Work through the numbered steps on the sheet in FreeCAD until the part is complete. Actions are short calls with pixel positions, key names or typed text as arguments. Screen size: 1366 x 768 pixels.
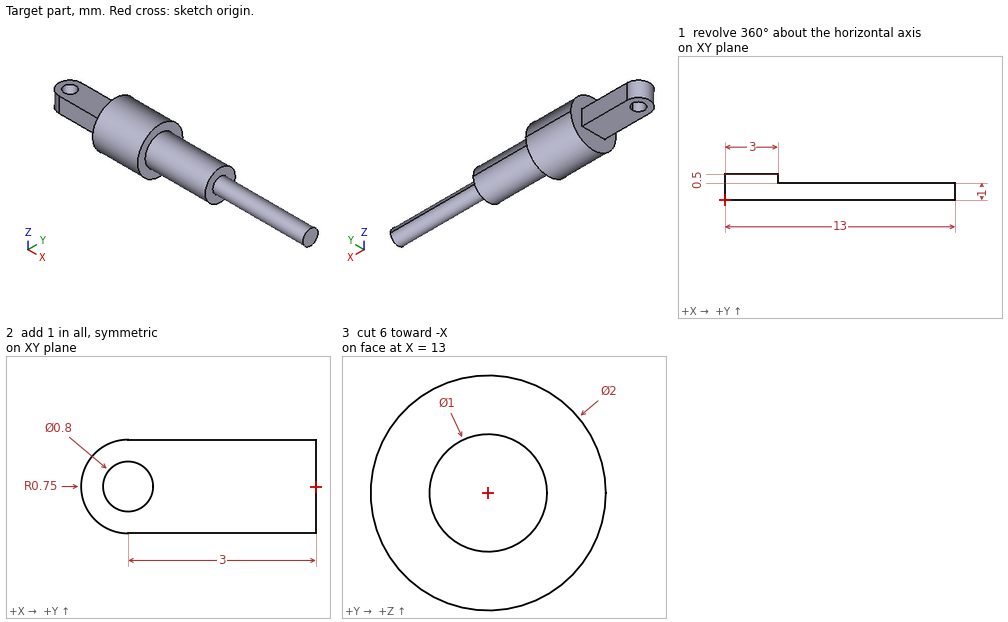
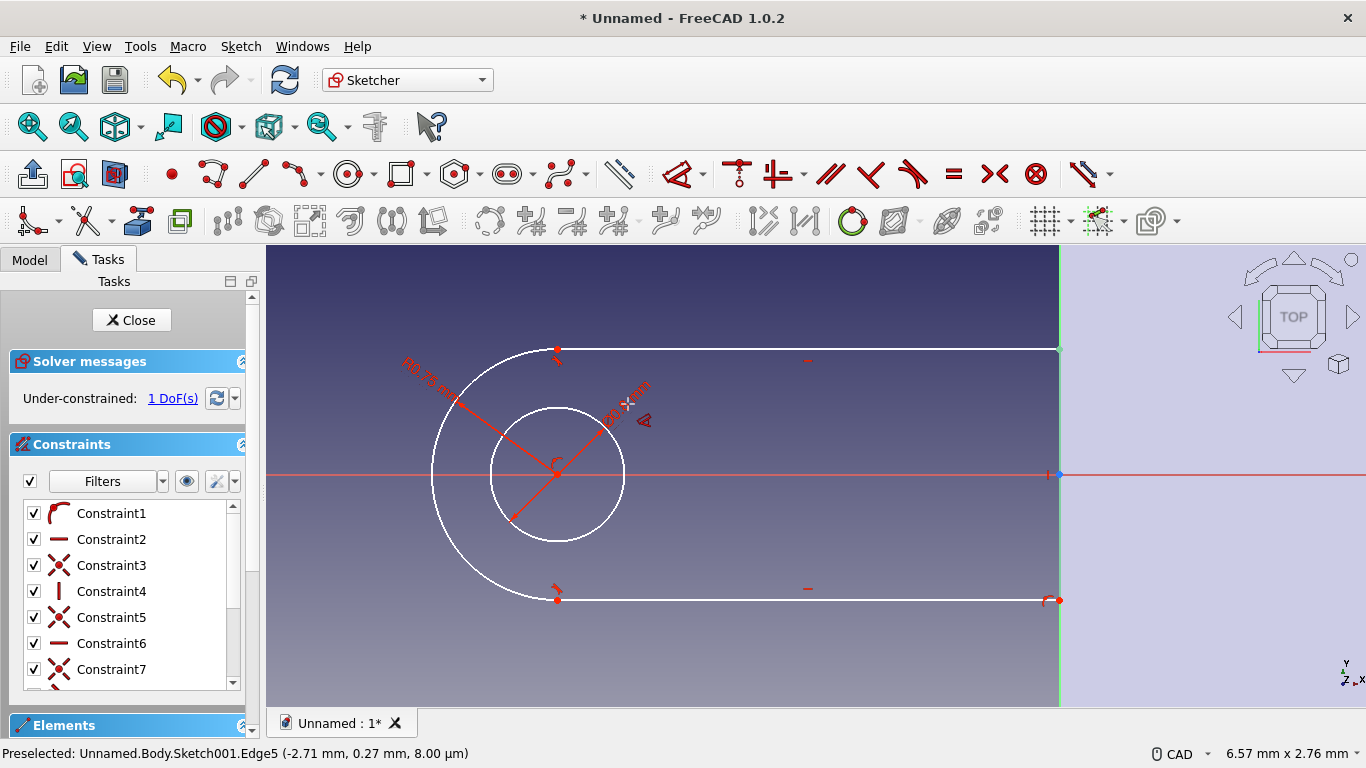
click(708, 600)
click(809, 634)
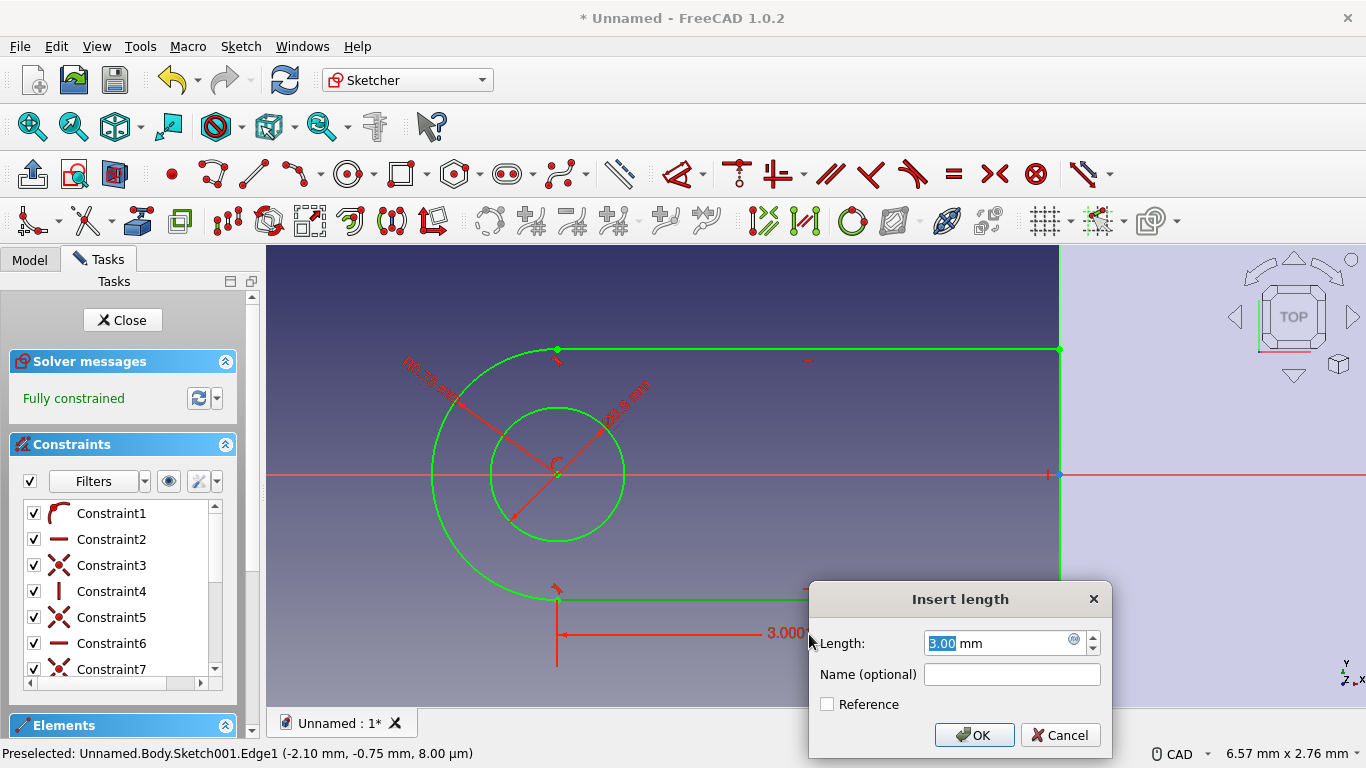
text(3)
key(Return)
key(Escape)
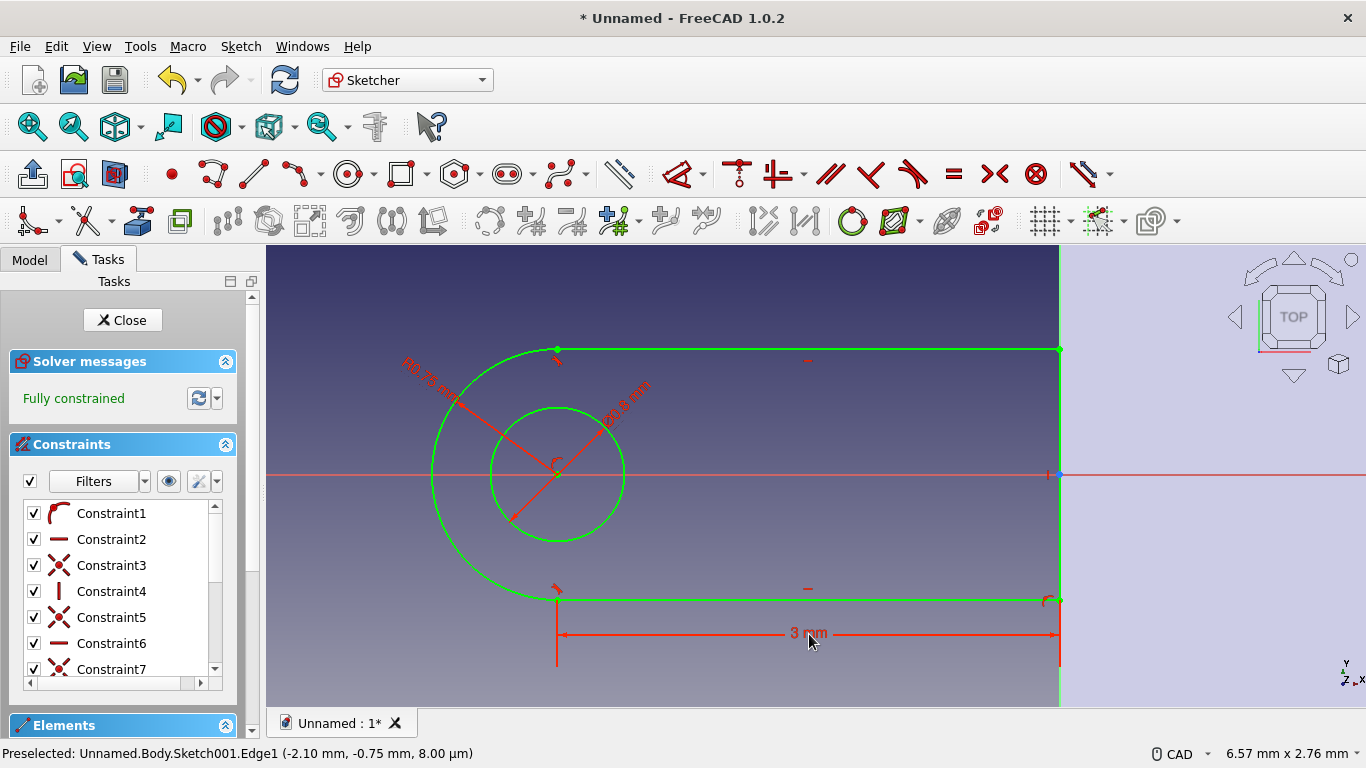
click(123, 320)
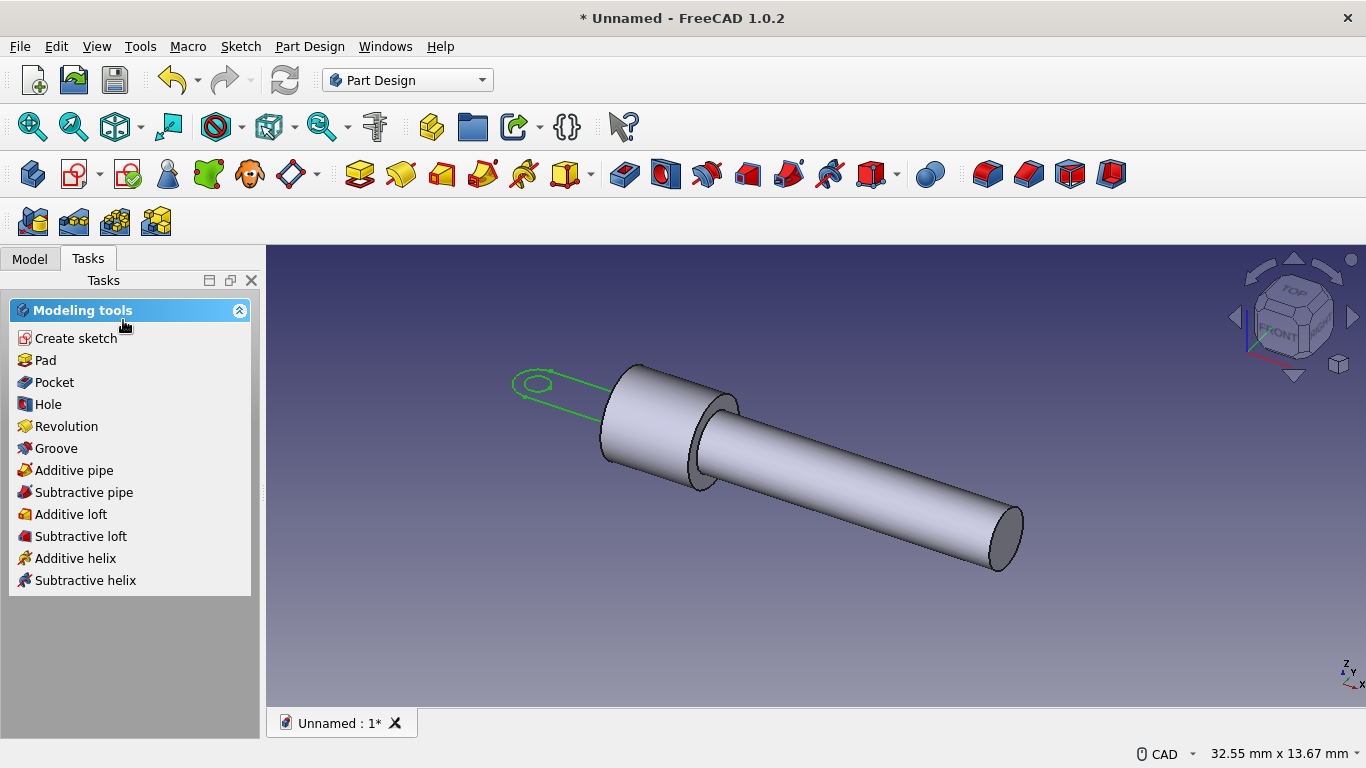
click(360, 174)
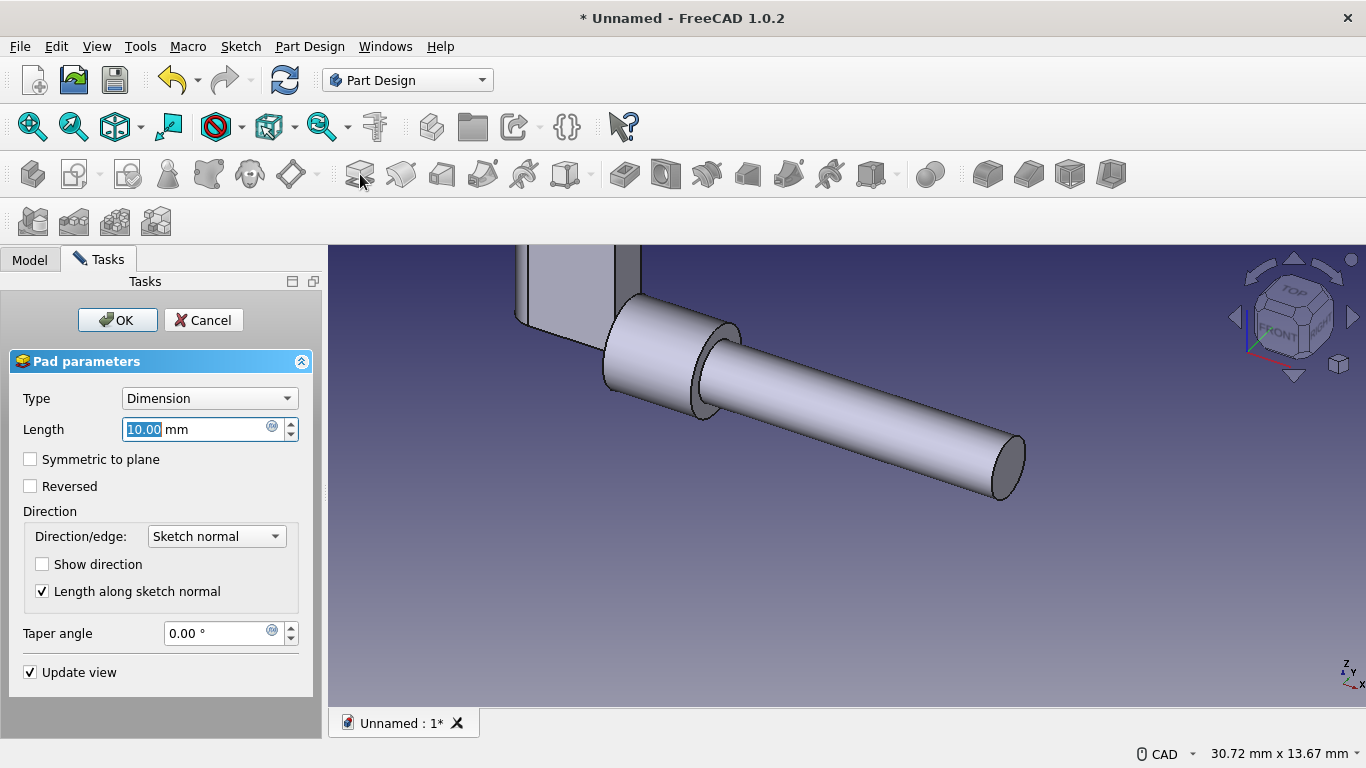
text(1)
key(Tab)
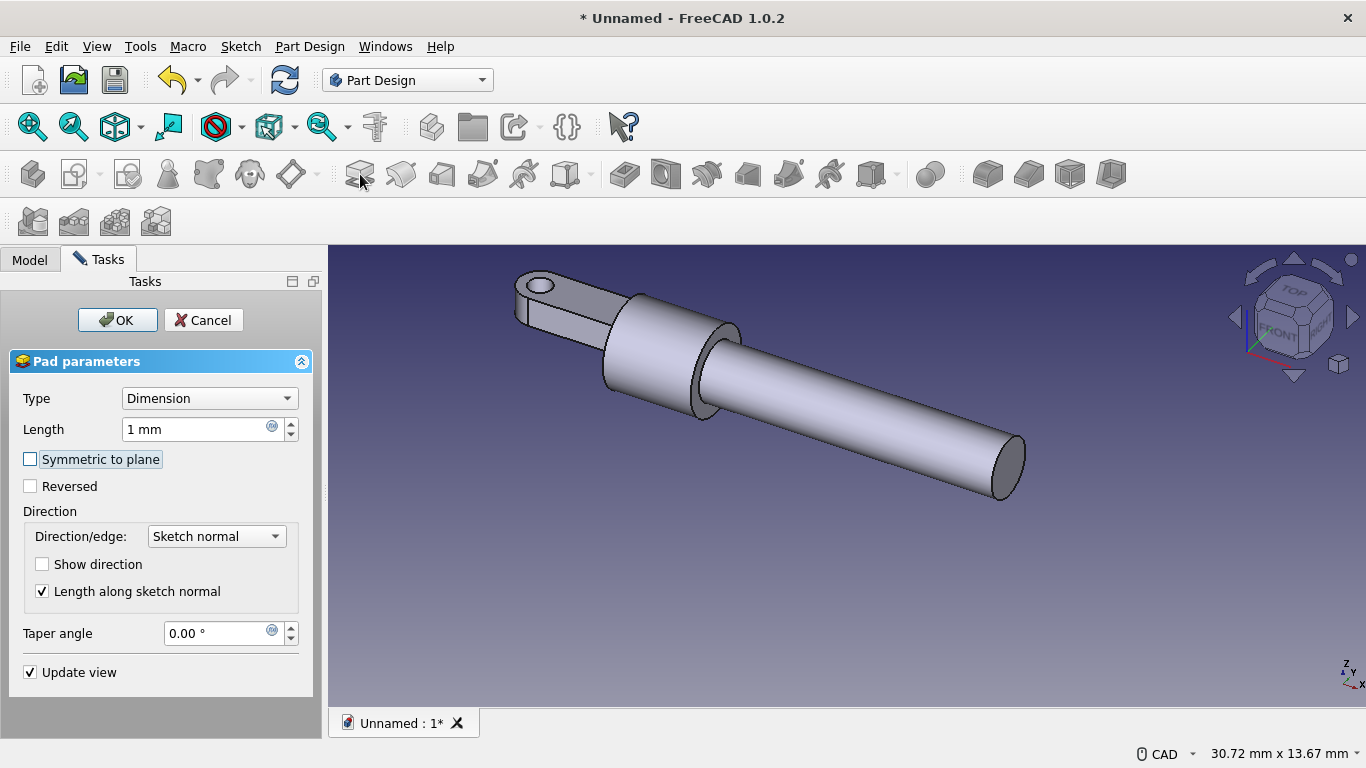
click(31, 459)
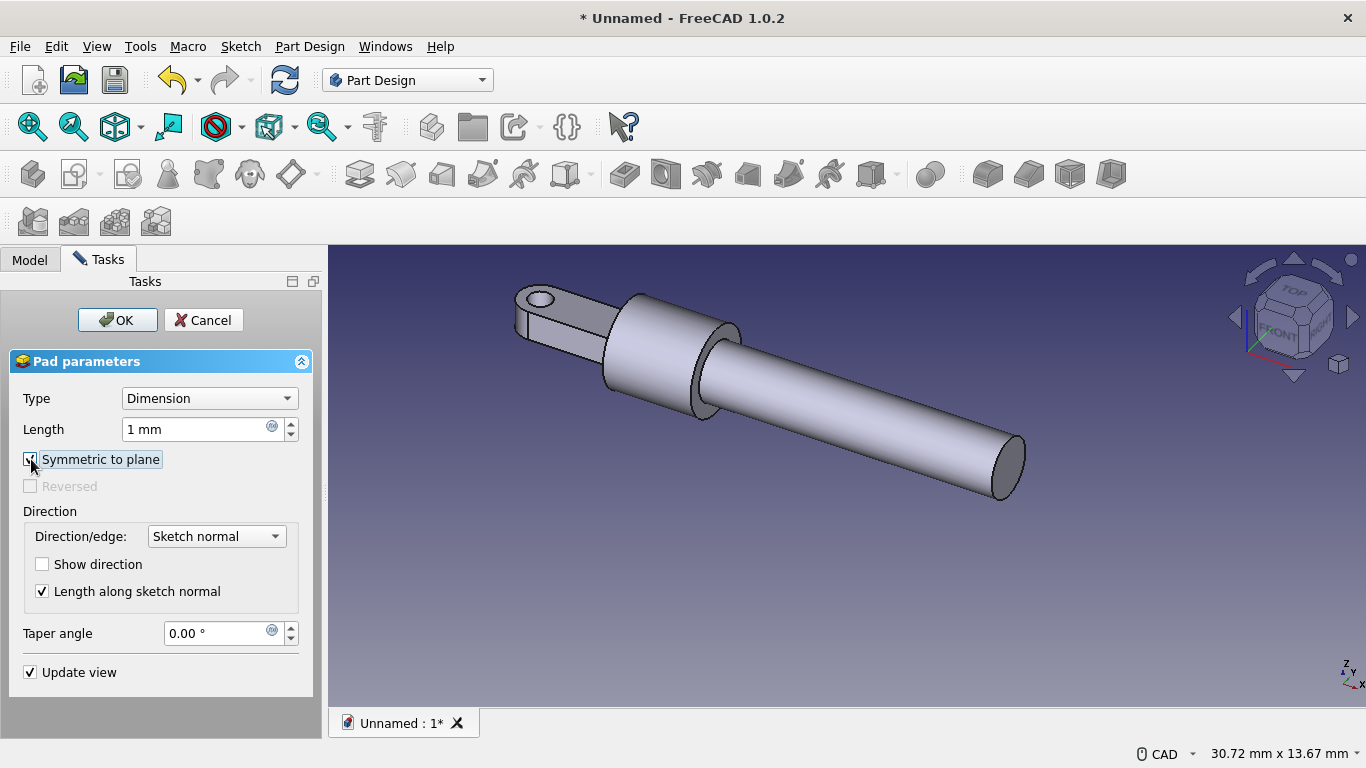
click(118, 320)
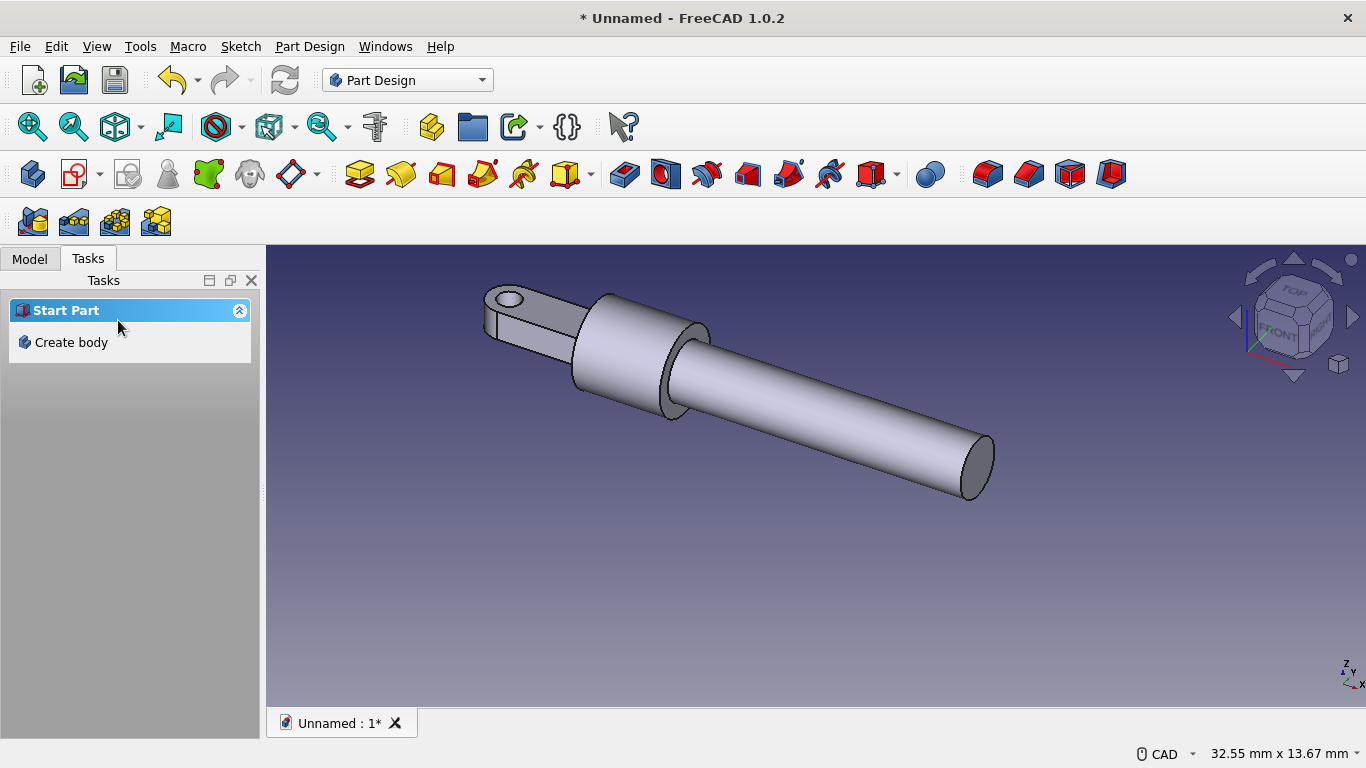
click(33, 128)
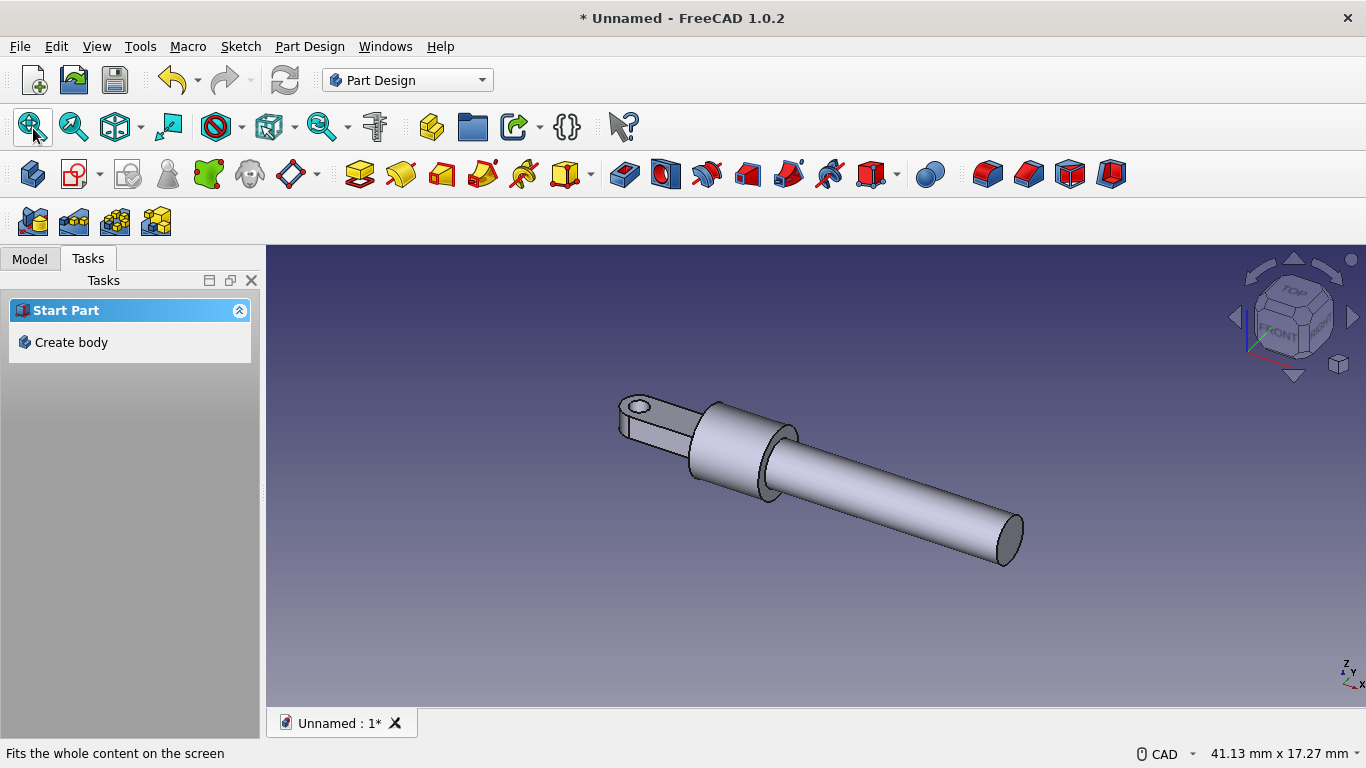
click(1010, 539)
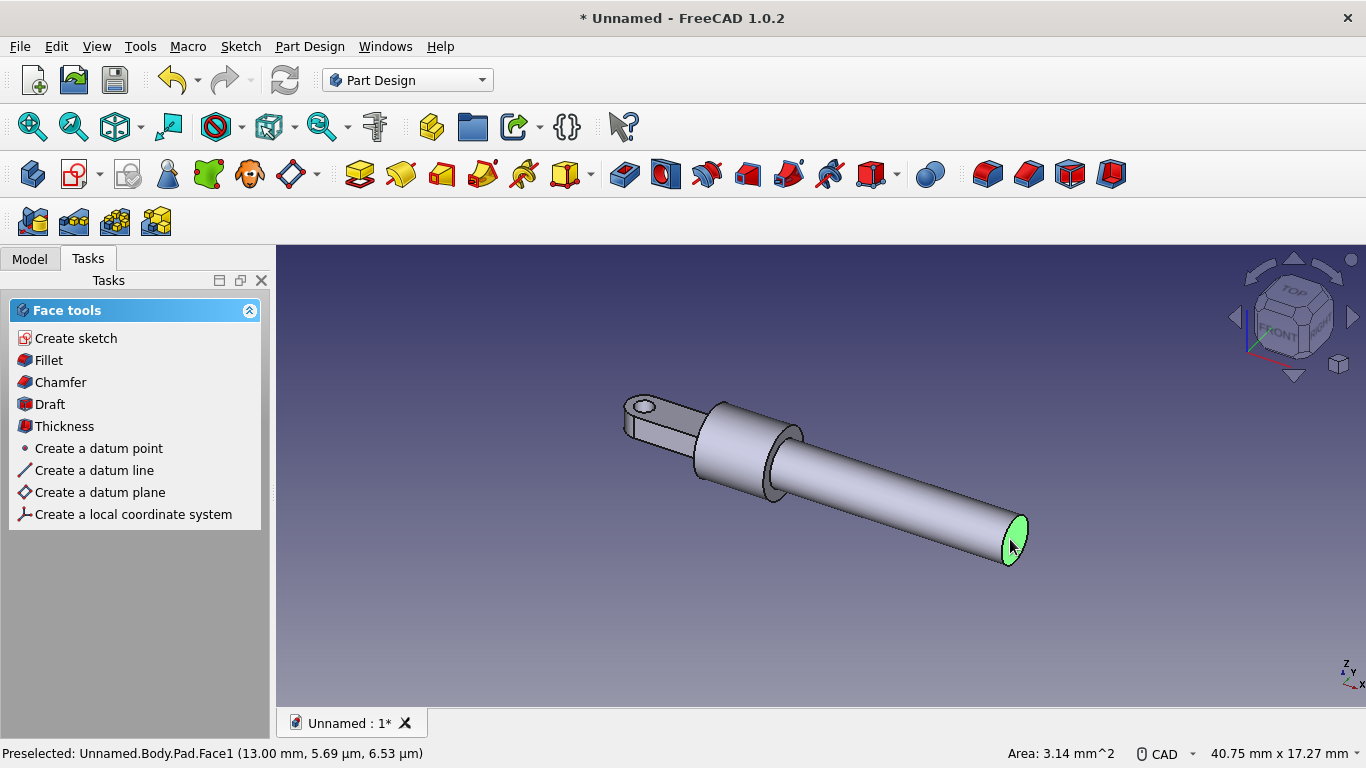
click(74, 174)